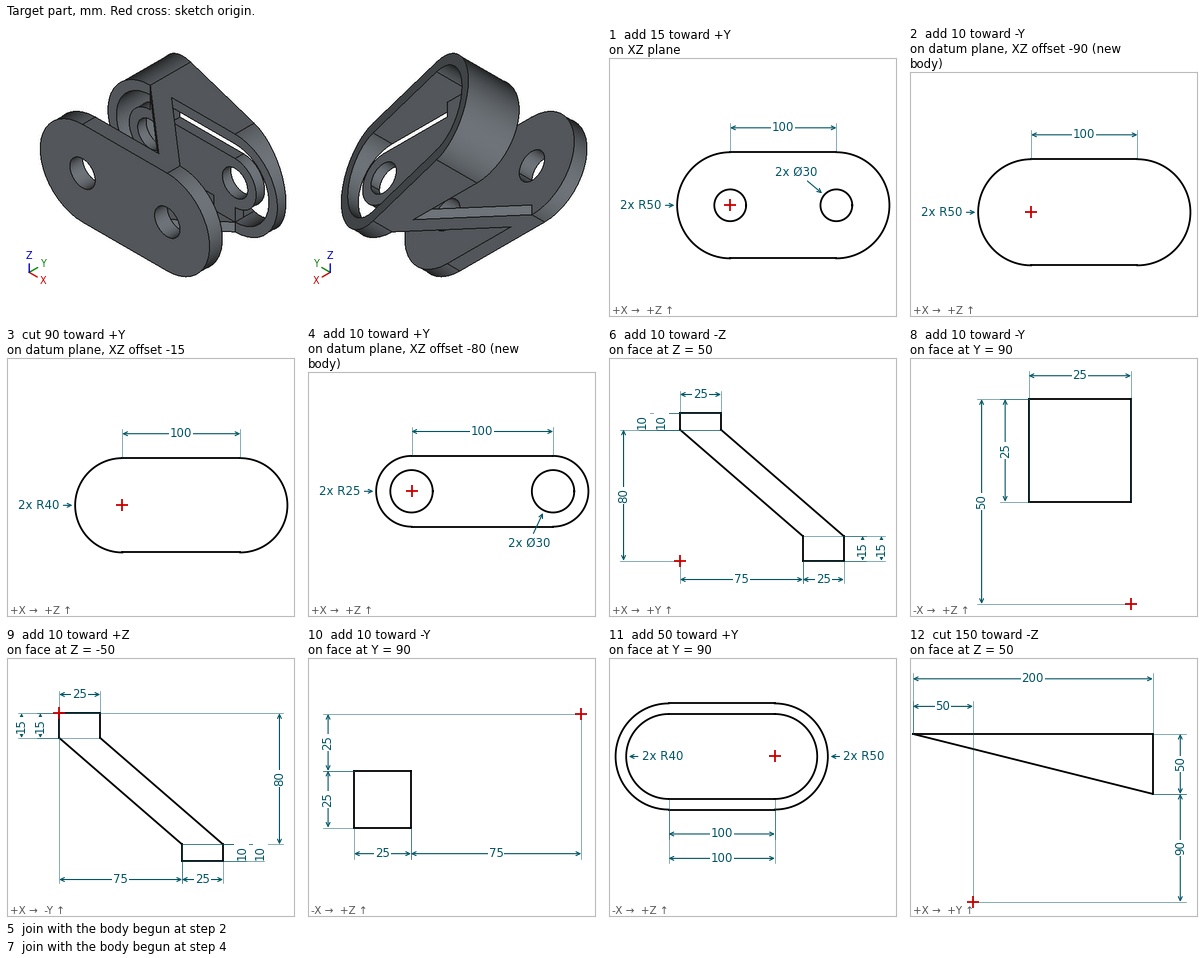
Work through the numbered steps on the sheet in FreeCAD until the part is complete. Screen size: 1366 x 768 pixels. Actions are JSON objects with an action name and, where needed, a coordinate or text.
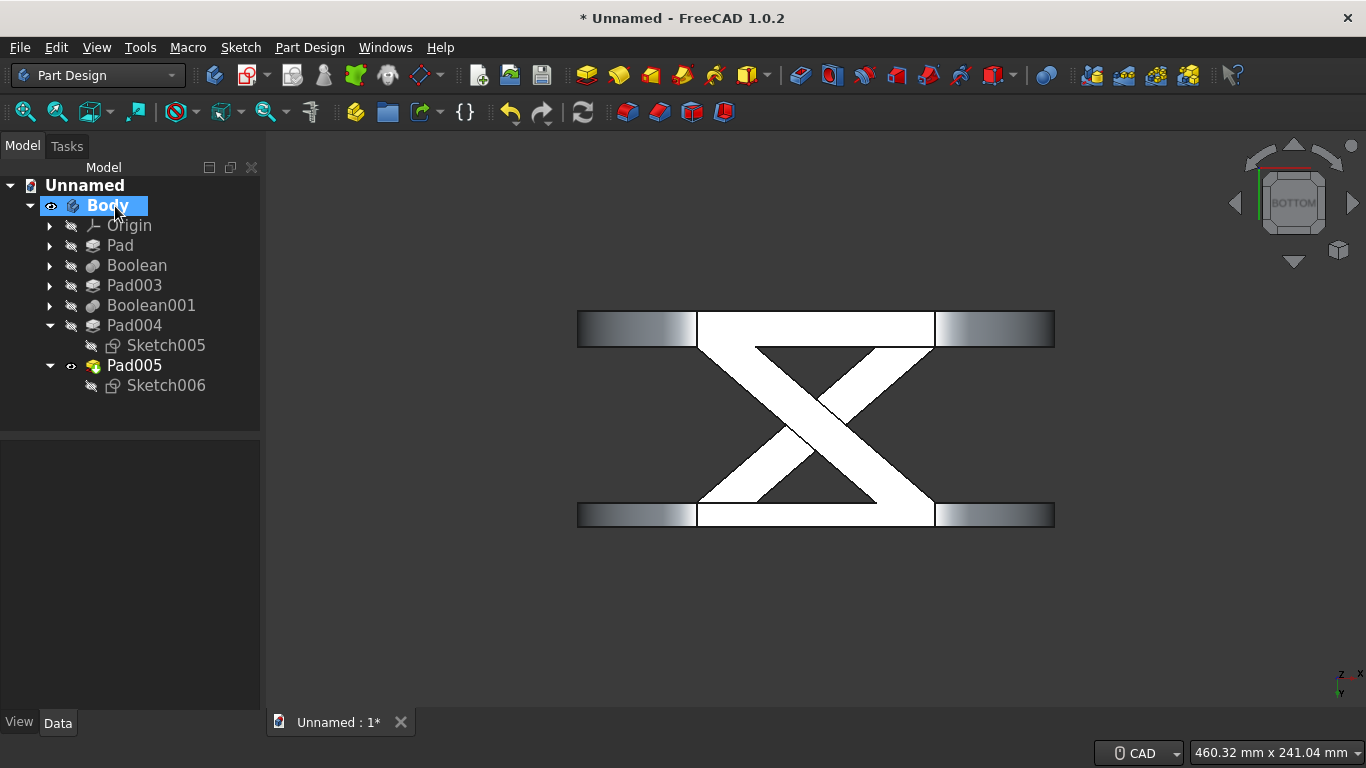
{"action": "left_click", "coordinate": [26, 112]}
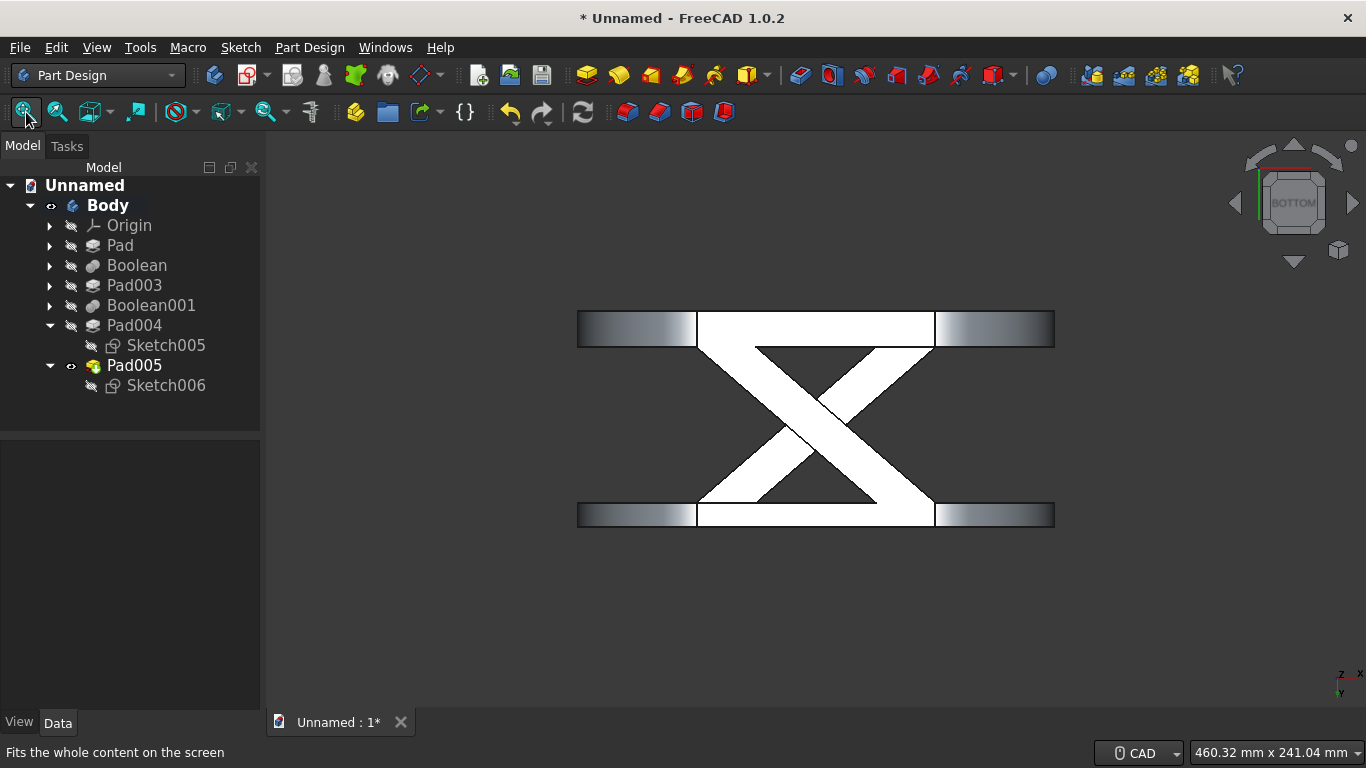
{"action": "key", "text": "4"}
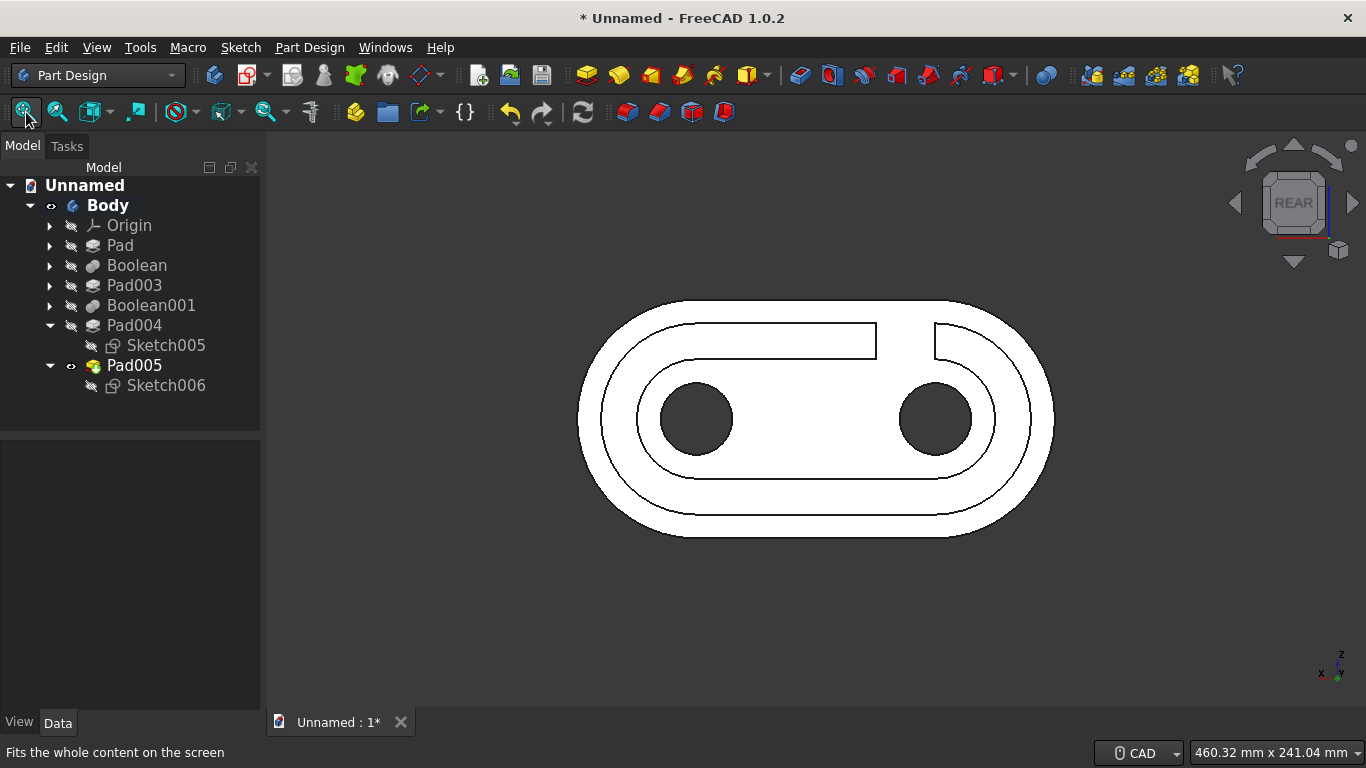
{"action": "left_click", "coordinate": [26, 112]}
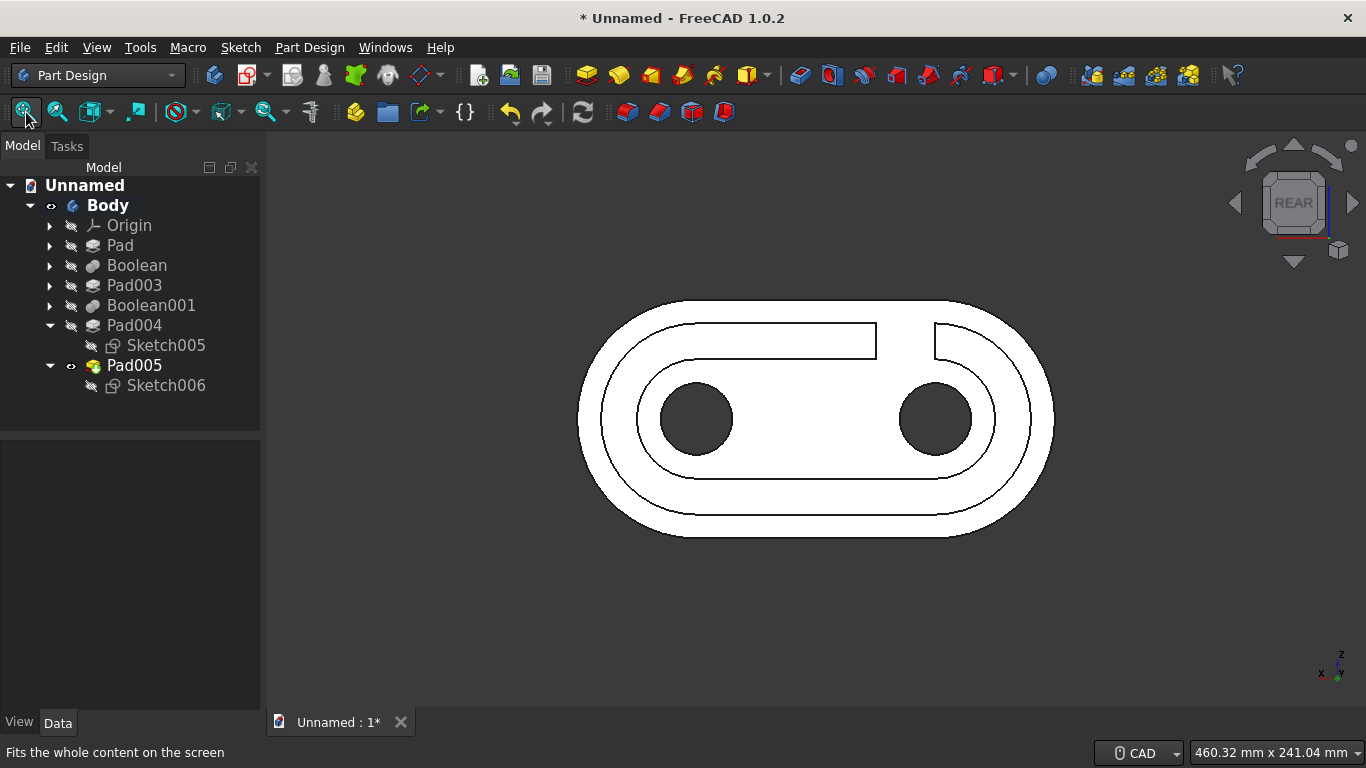
{"action": "left_click", "coordinate": [816, 418]}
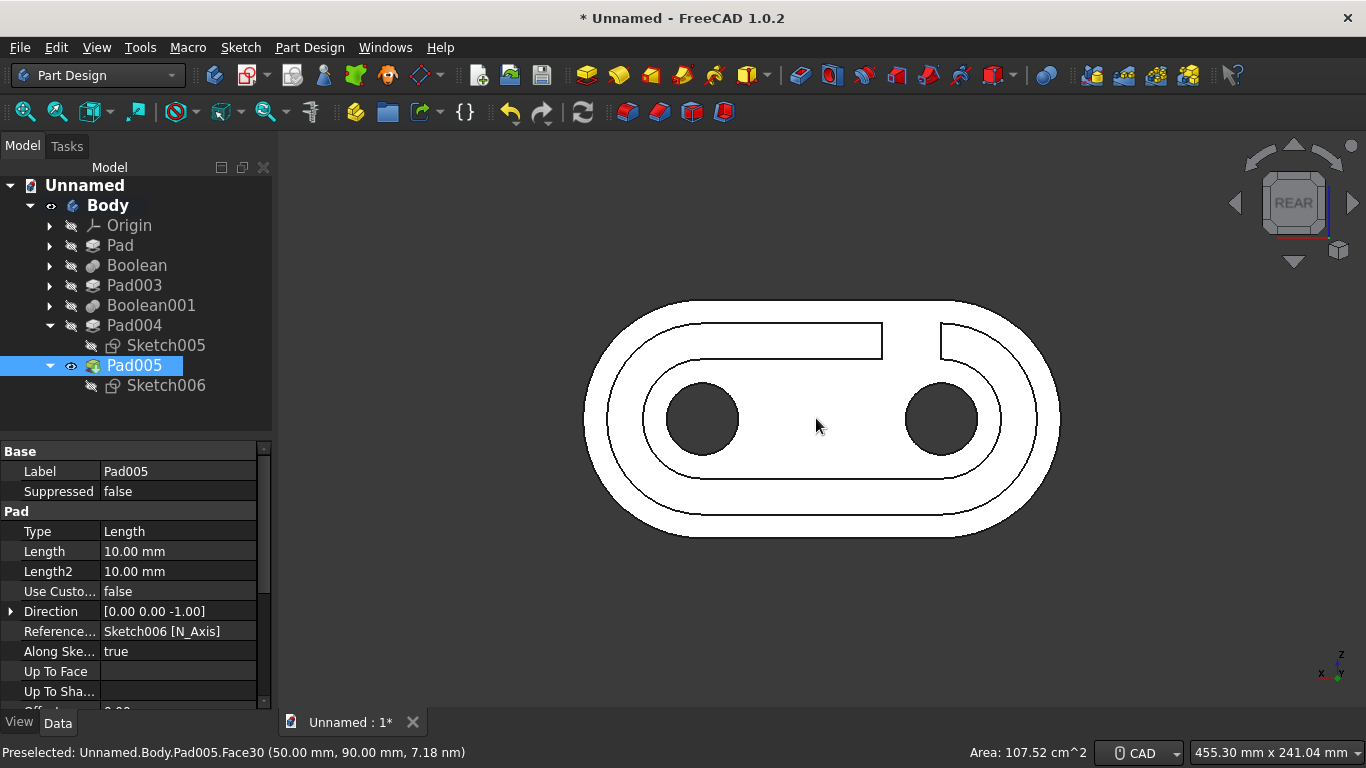
{"action": "left_click", "coordinate": [248, 76]}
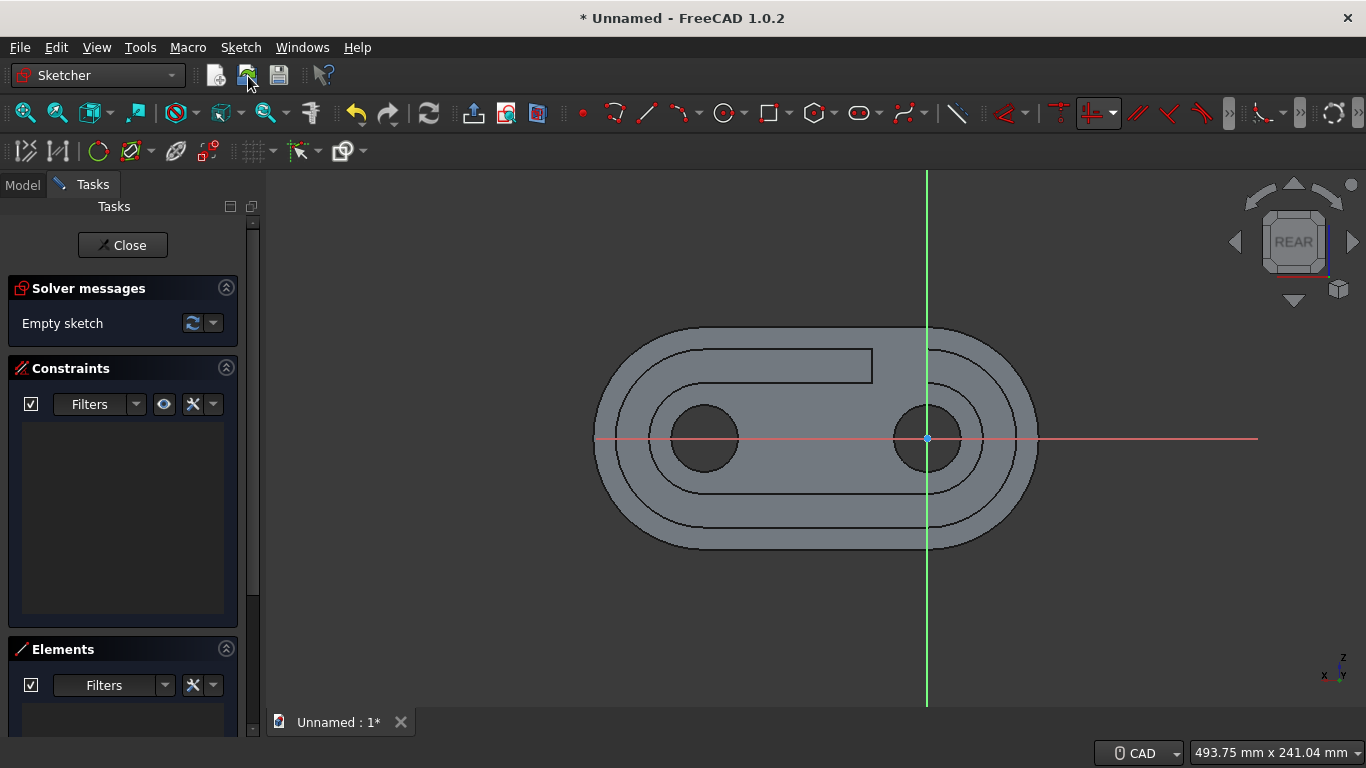
{"action": "scroll", "coordinate": [729, 539], "scroll_direction": "up", "scroll_amount": 9}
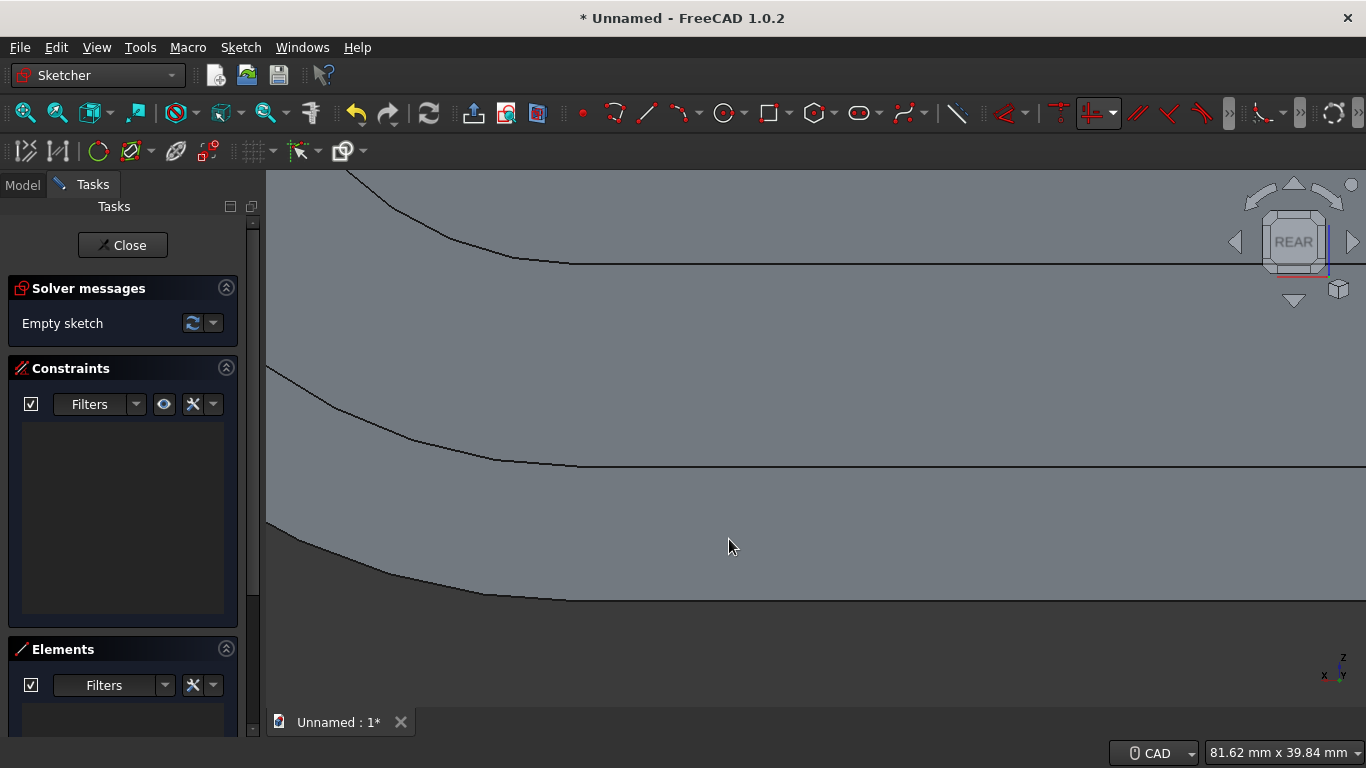
{"action": "left_click", "coordinate": [770, 114]}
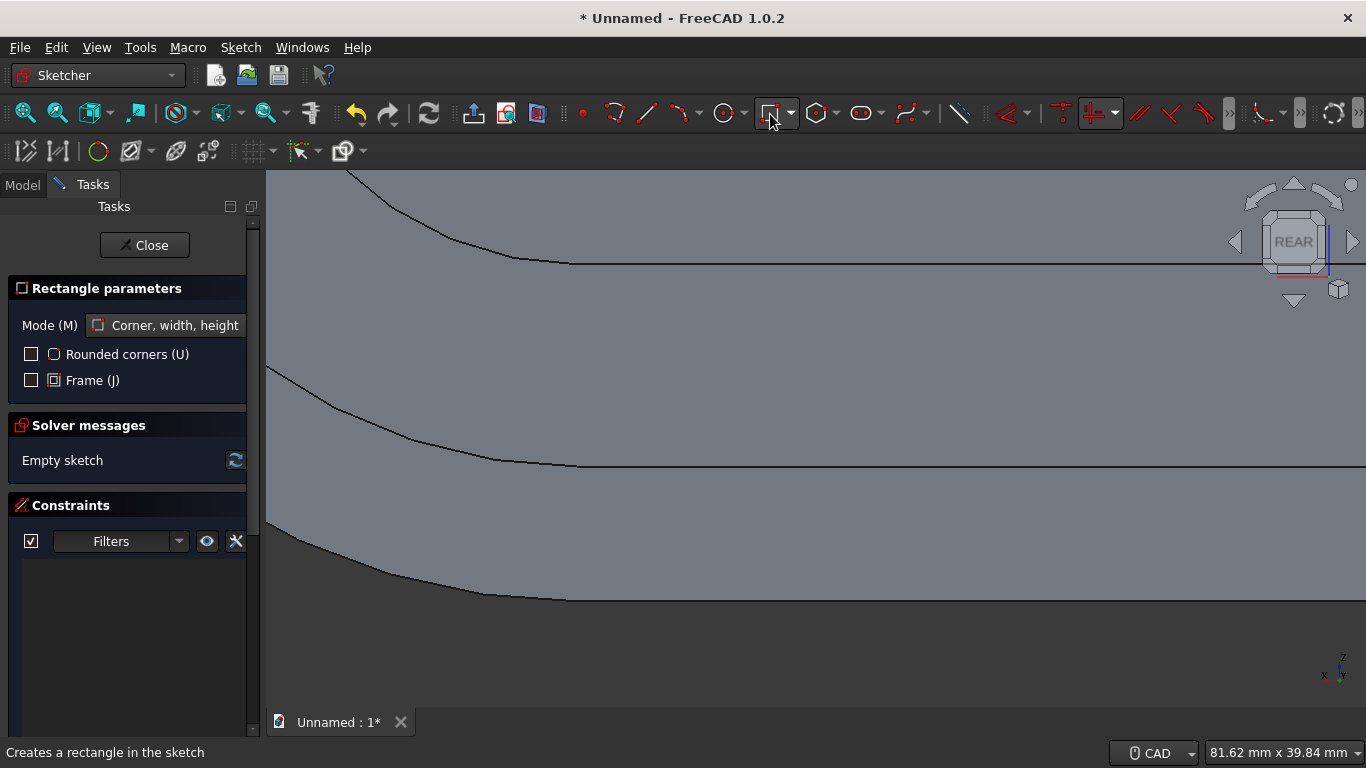
{"action": "left_click", "coordinate": [579, 264]}
{"action": "left_click", "coordinate": [916, 601]}
{"action": "key", "text": "Escape"}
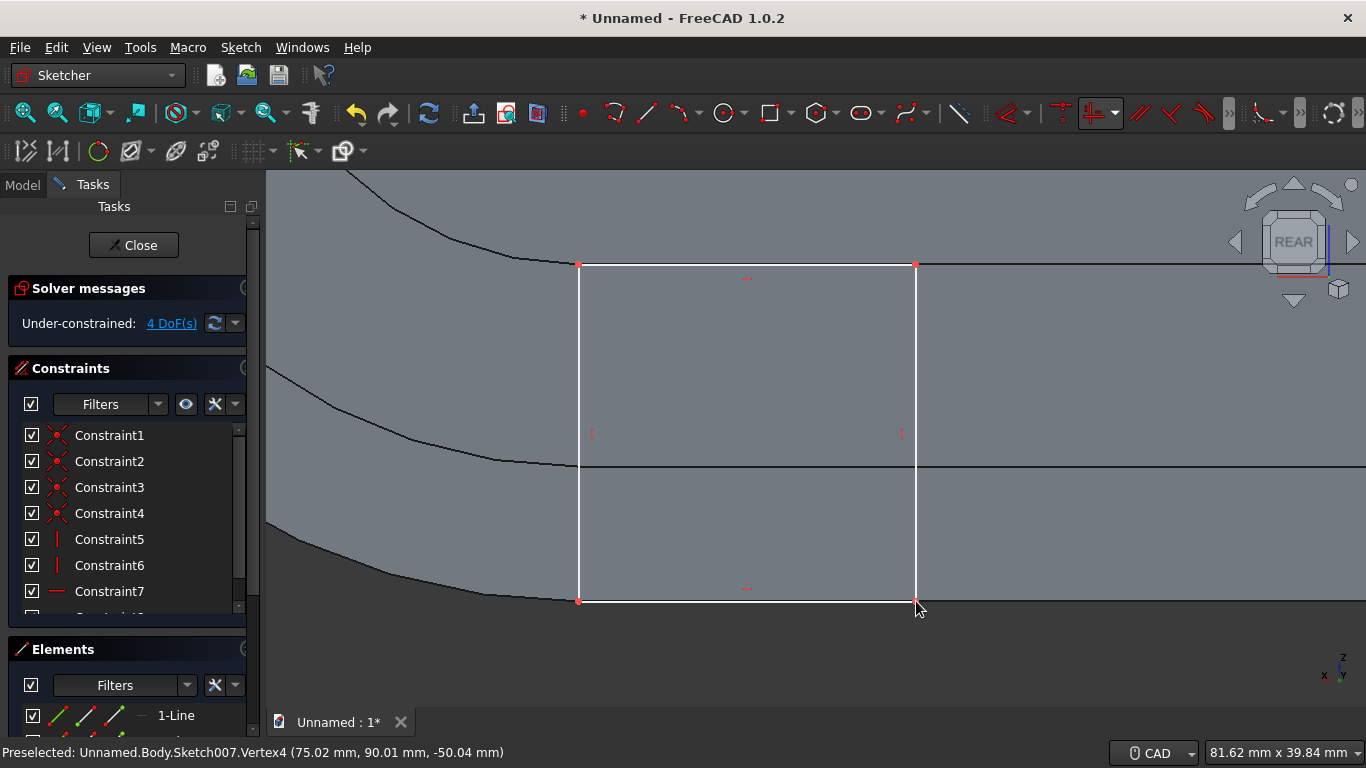
{"action": "left_click", "coordinate": [1006, 114]}